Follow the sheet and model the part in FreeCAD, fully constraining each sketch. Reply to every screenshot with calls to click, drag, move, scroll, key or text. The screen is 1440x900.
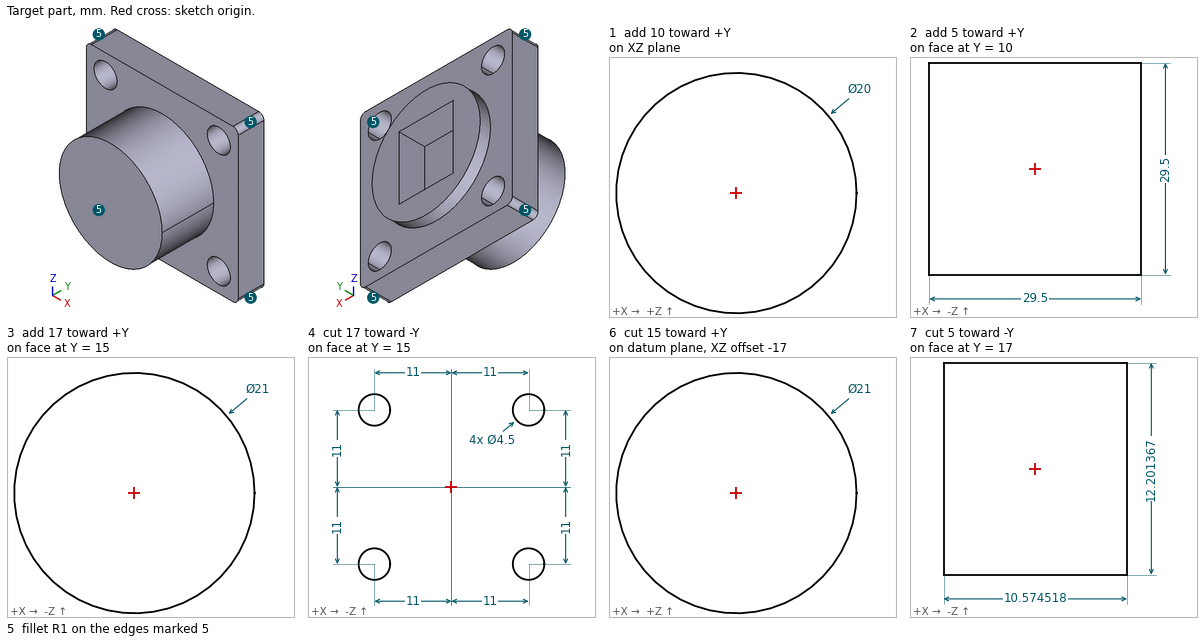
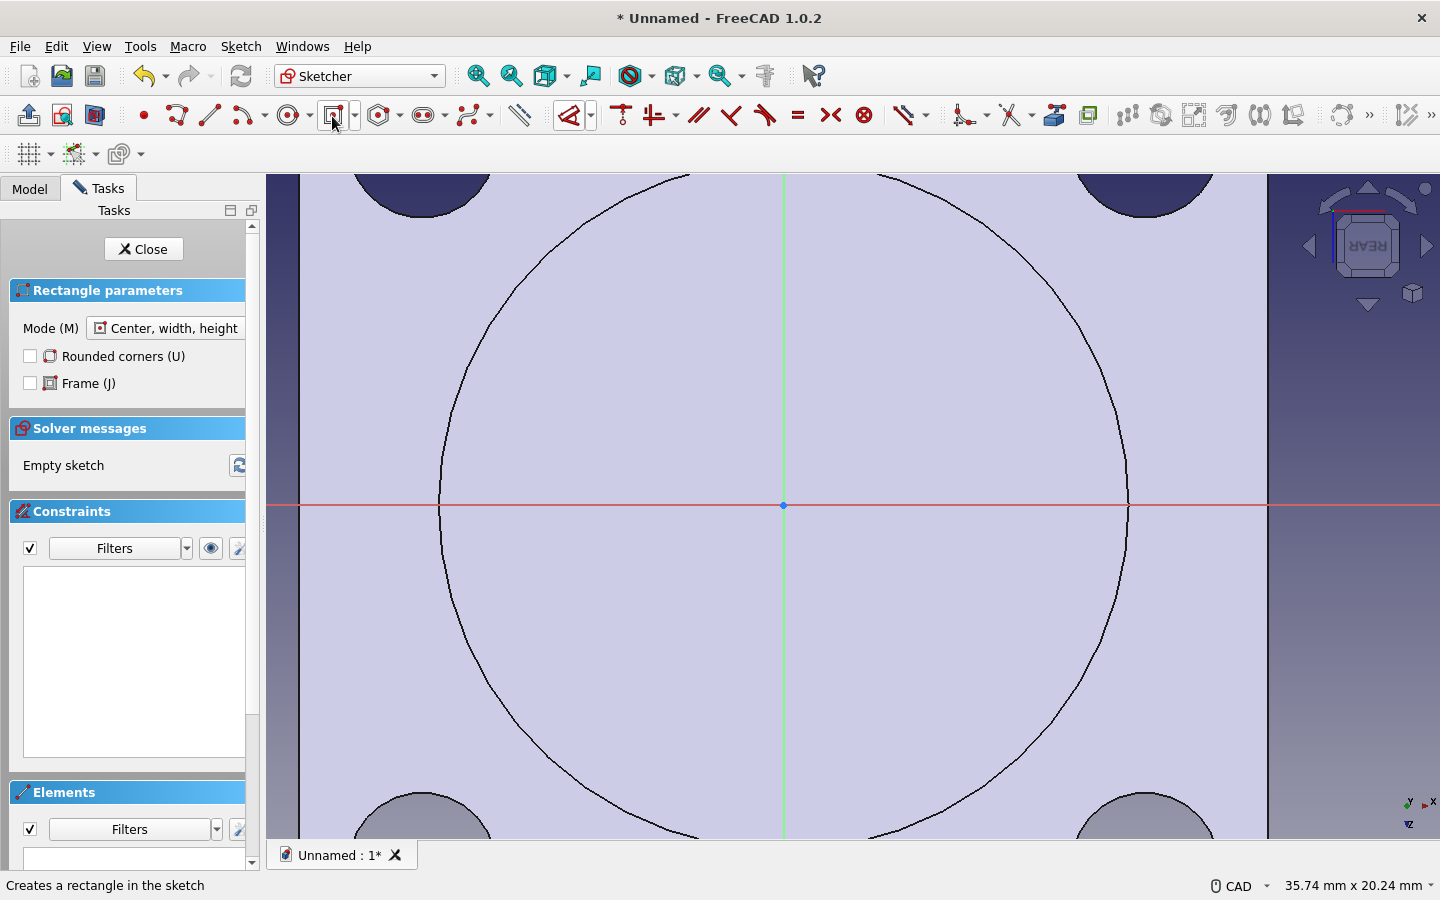
click(784, 505)
click(957, 305)
key(Escape)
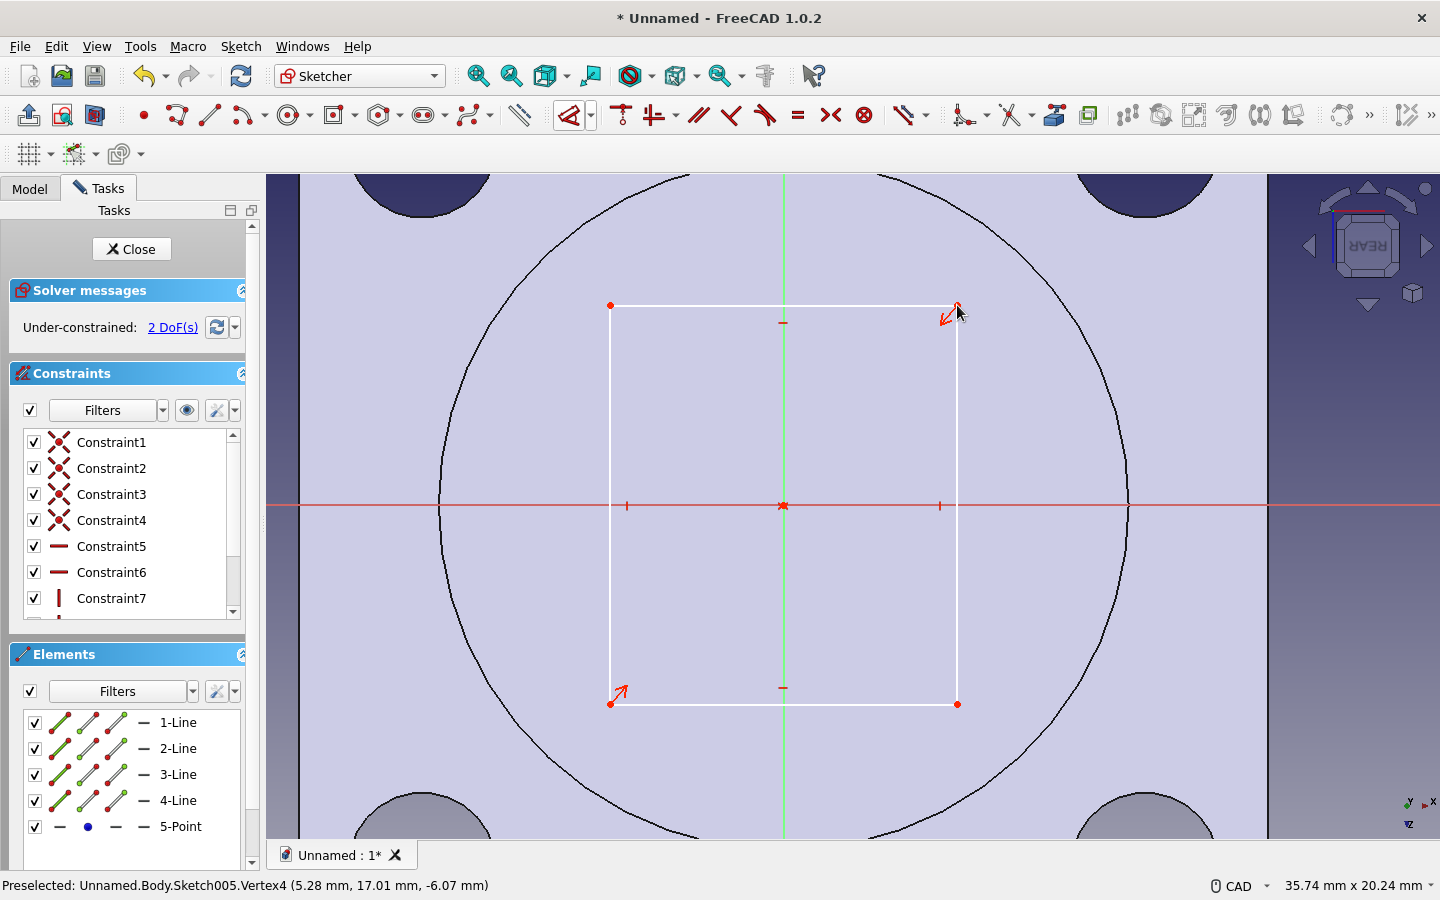
click(714, 705)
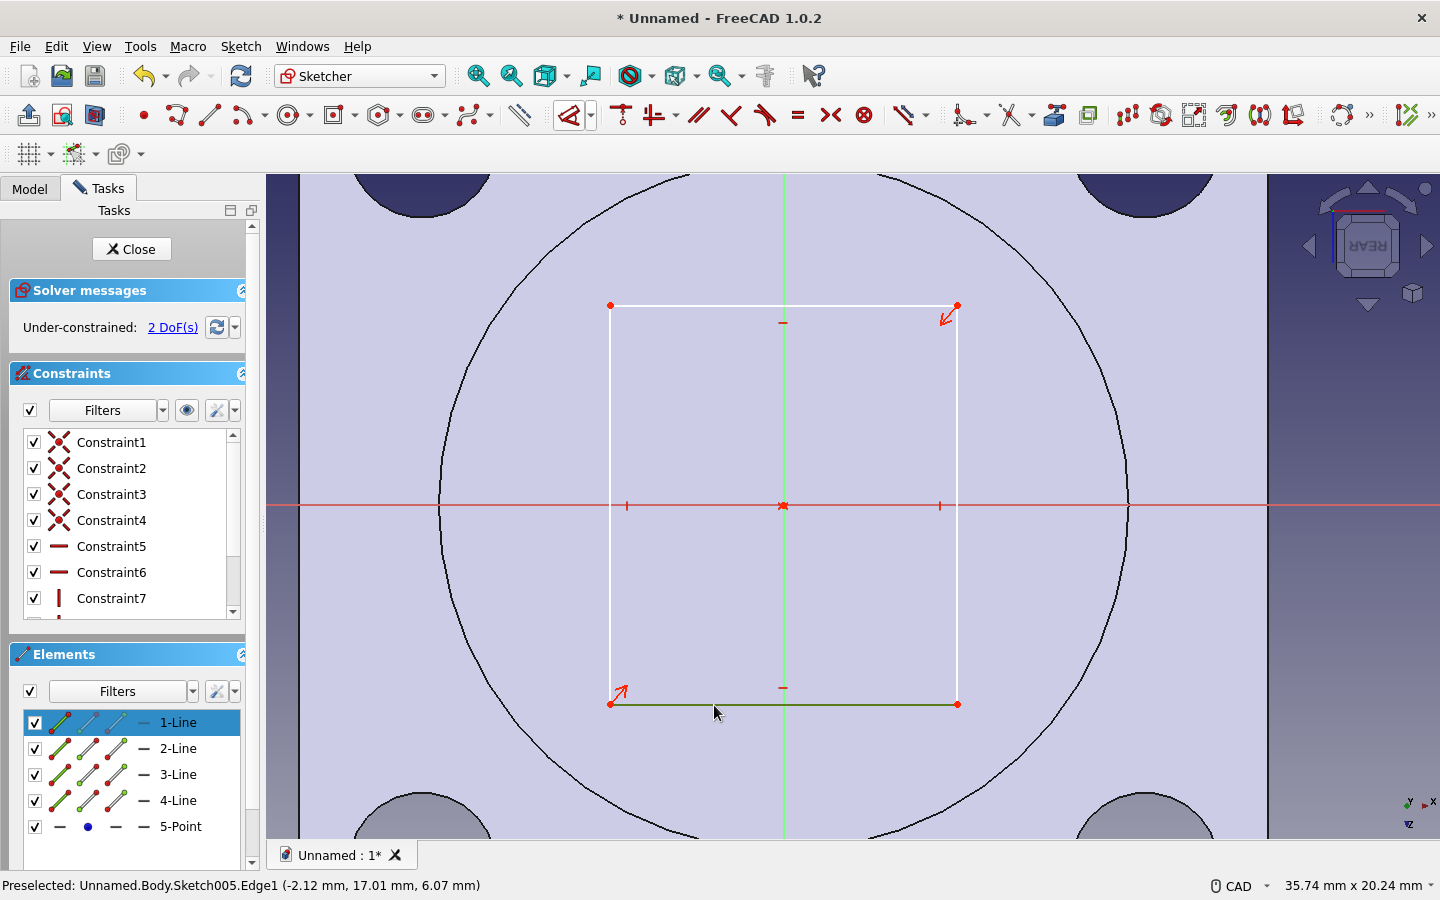
key(l)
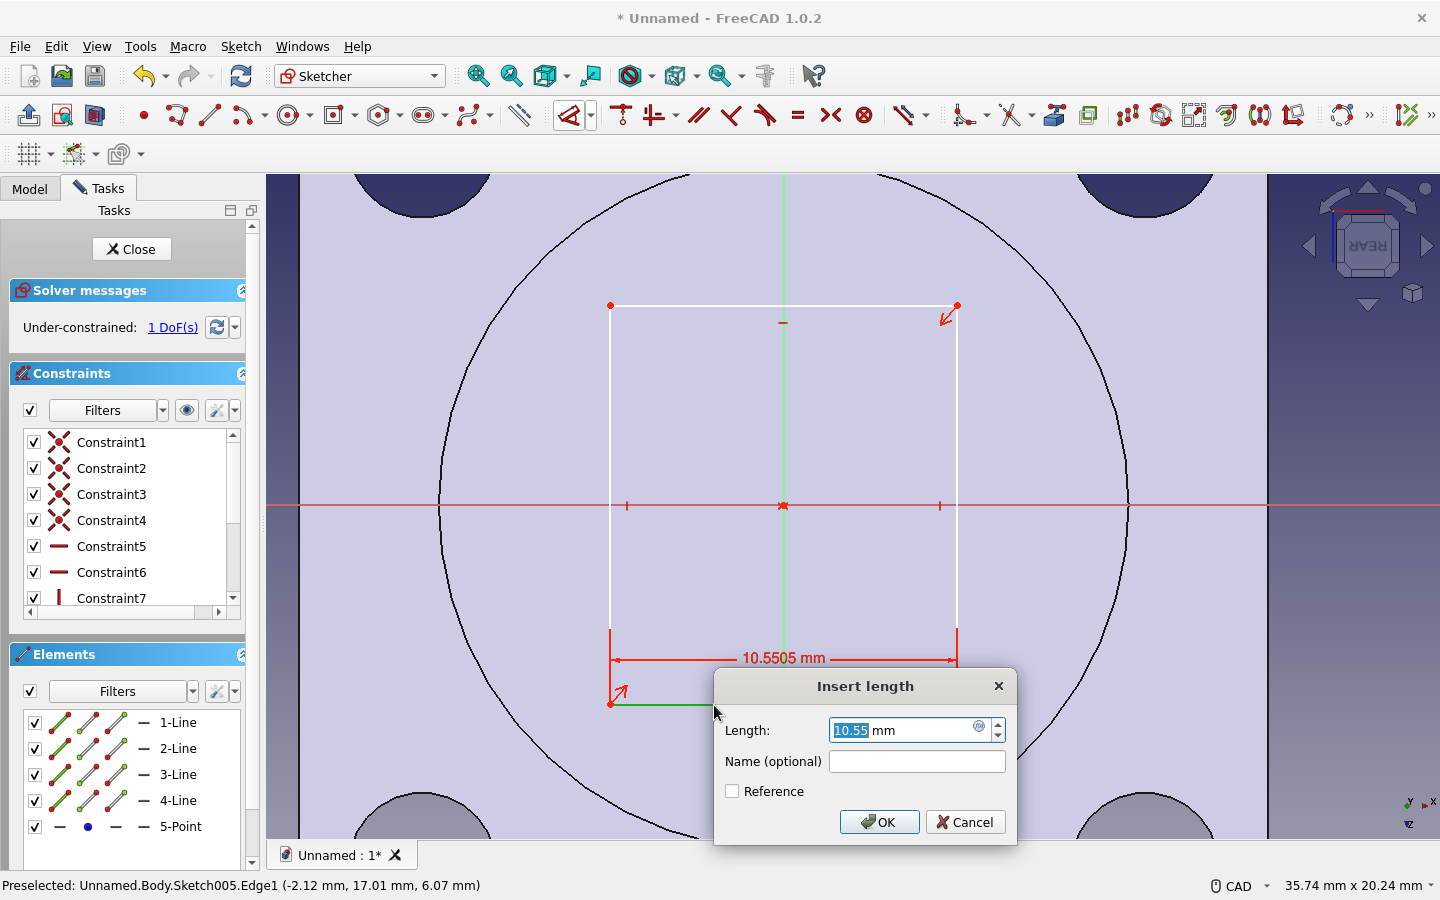
text(10.574518)
key(Return)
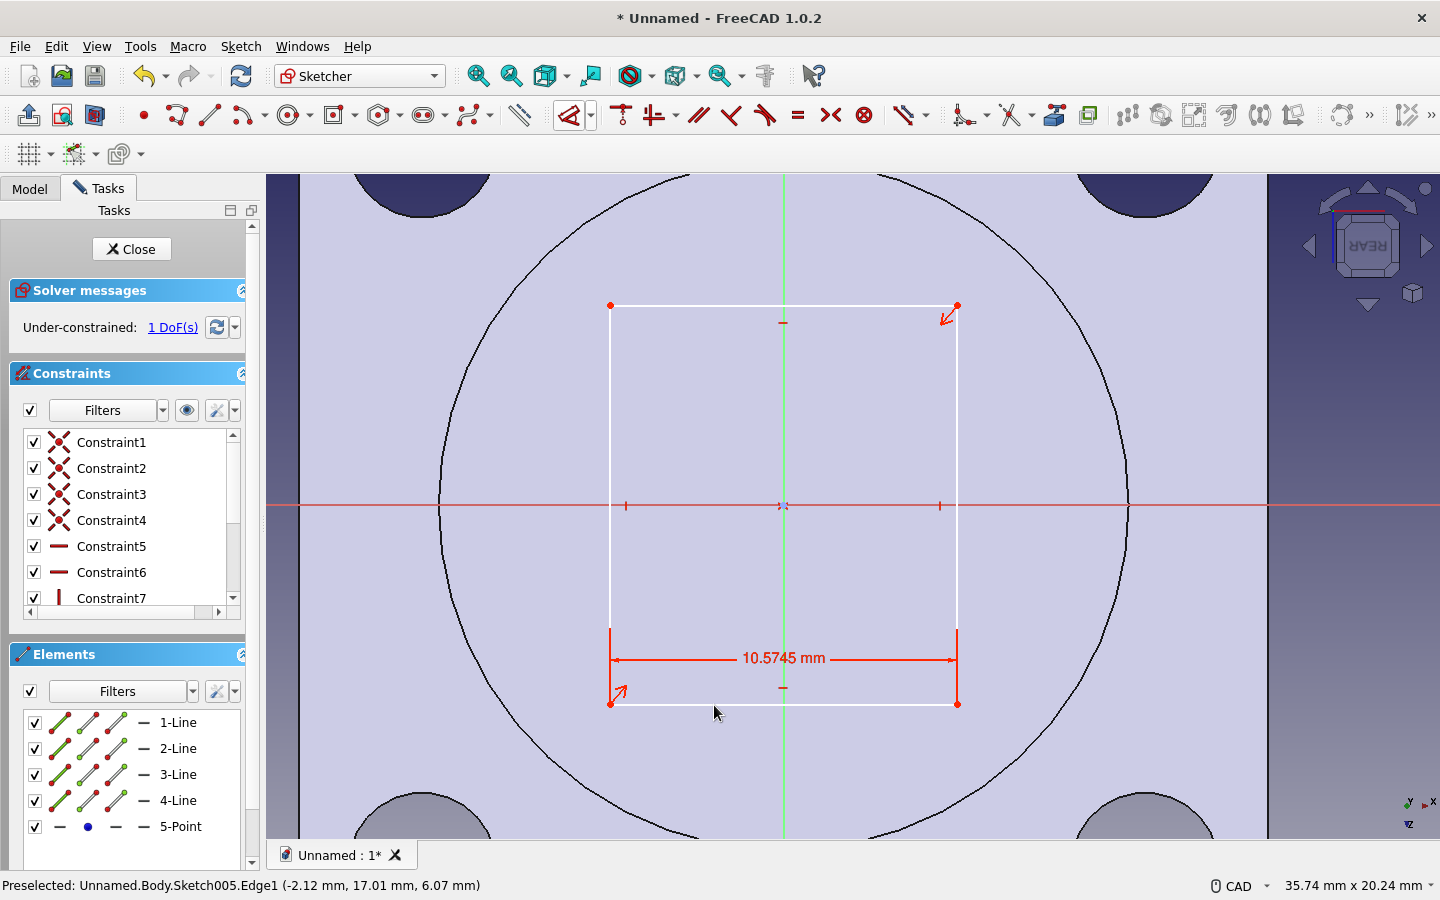
click(957, 585)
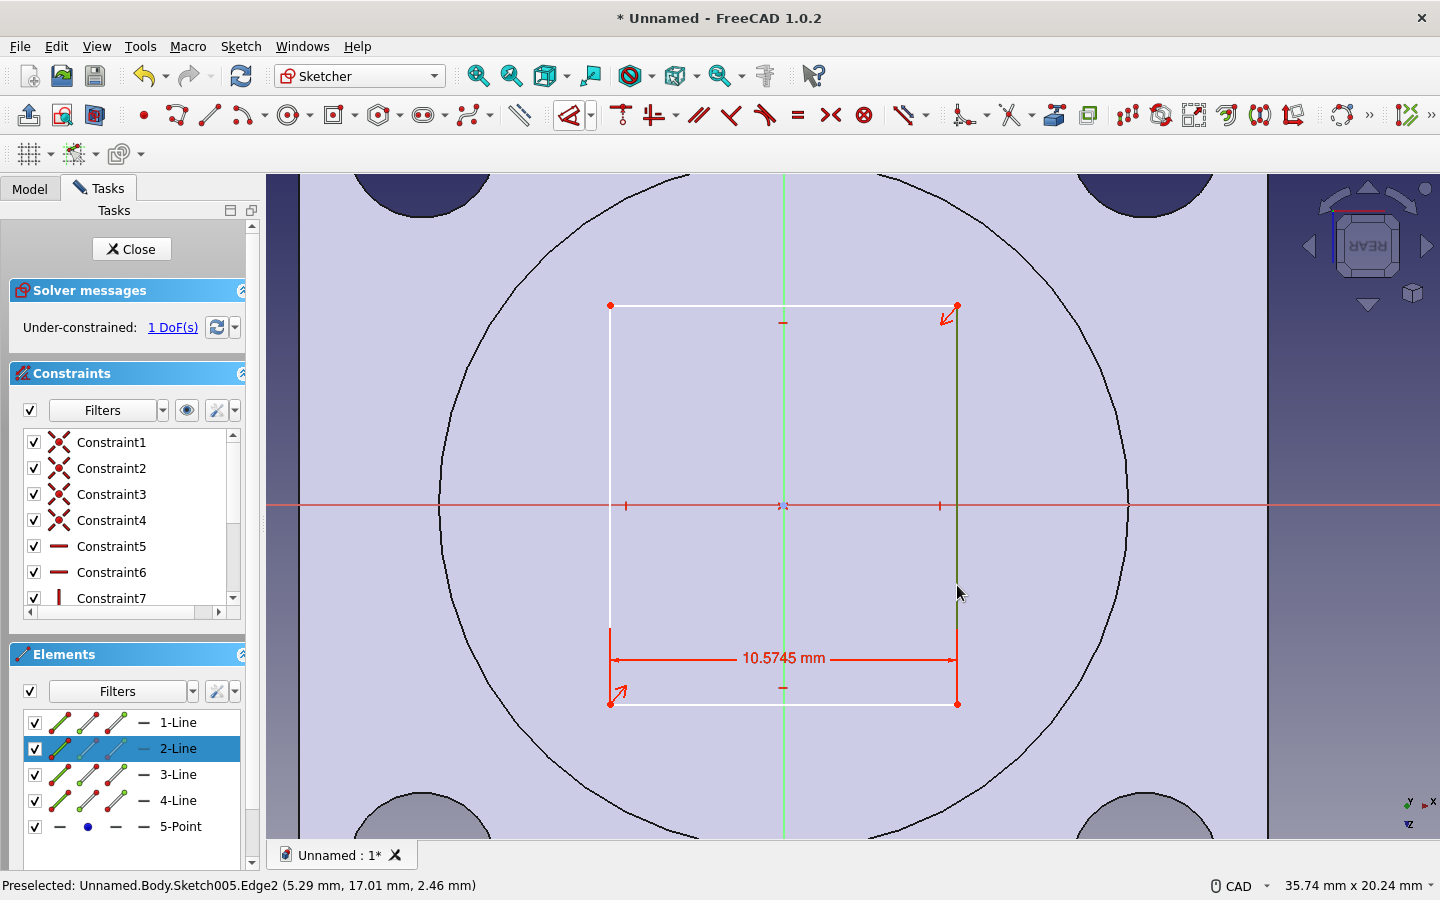
key(i)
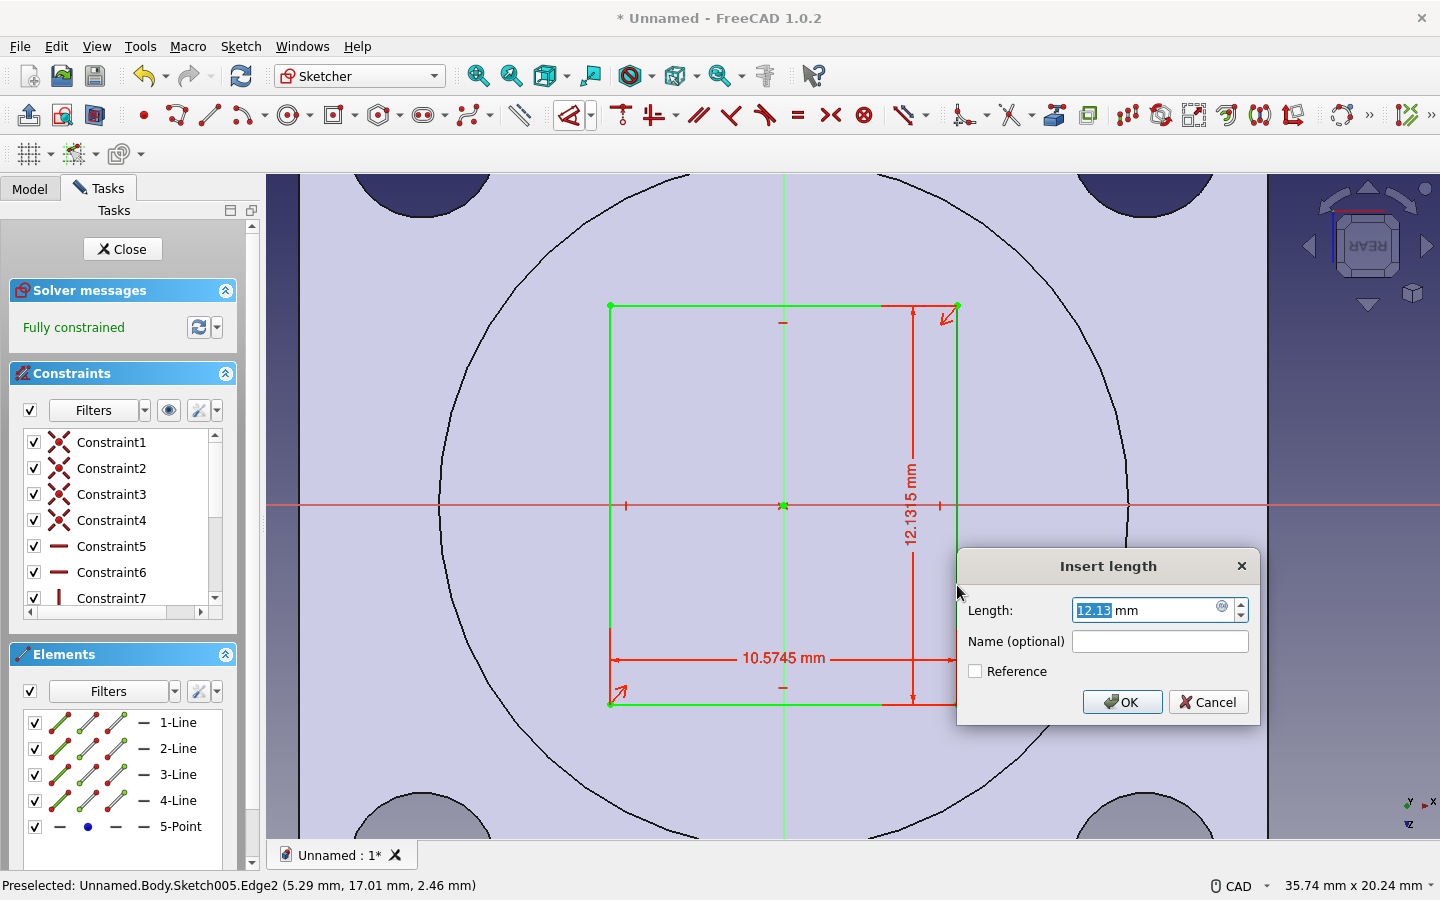
text(12.201367)
key(Return)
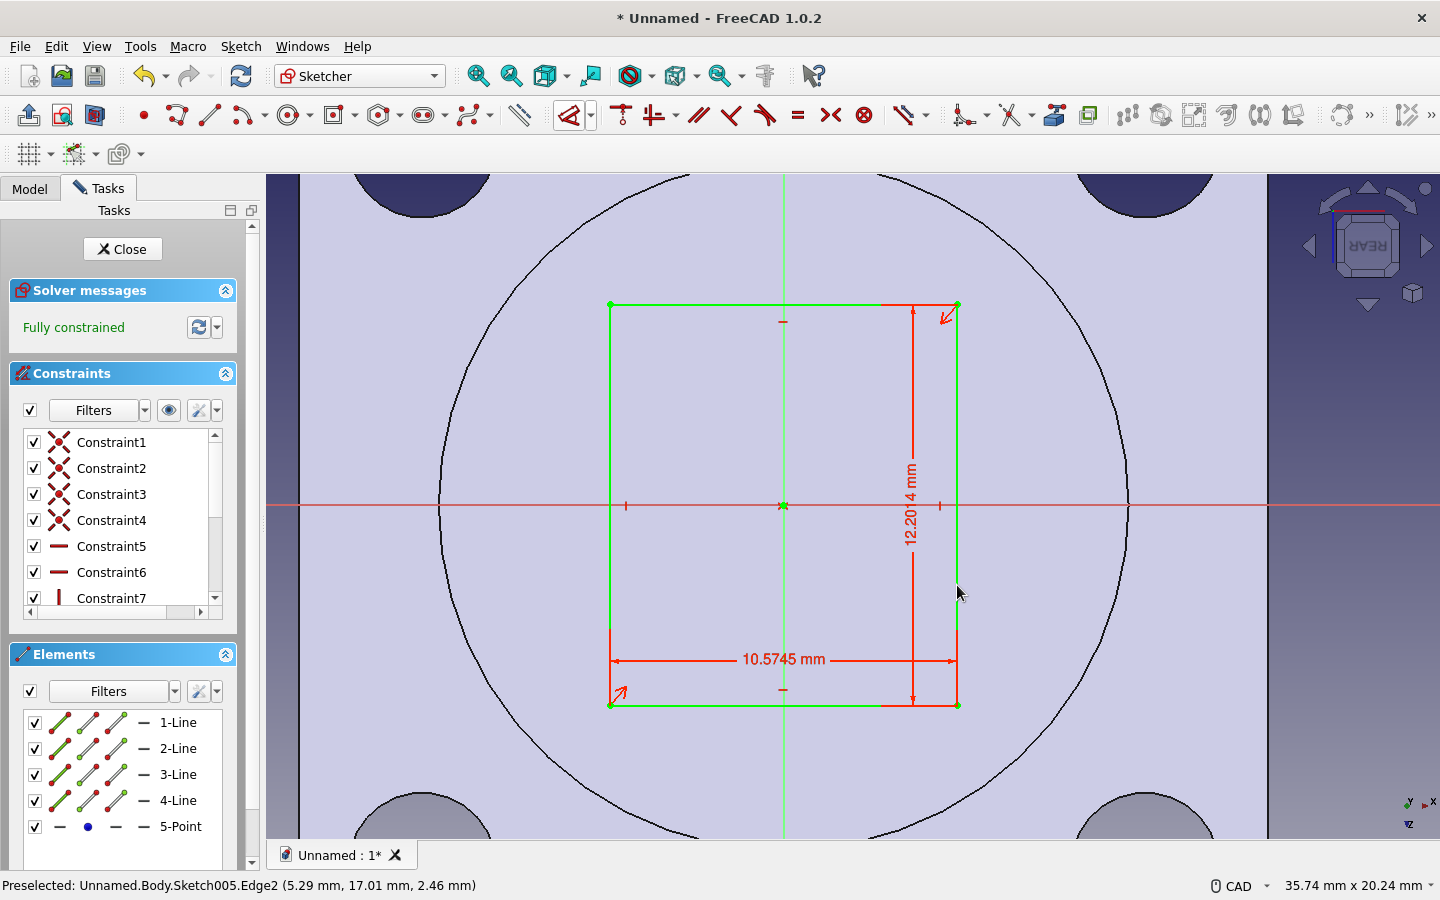
click(123, 249)